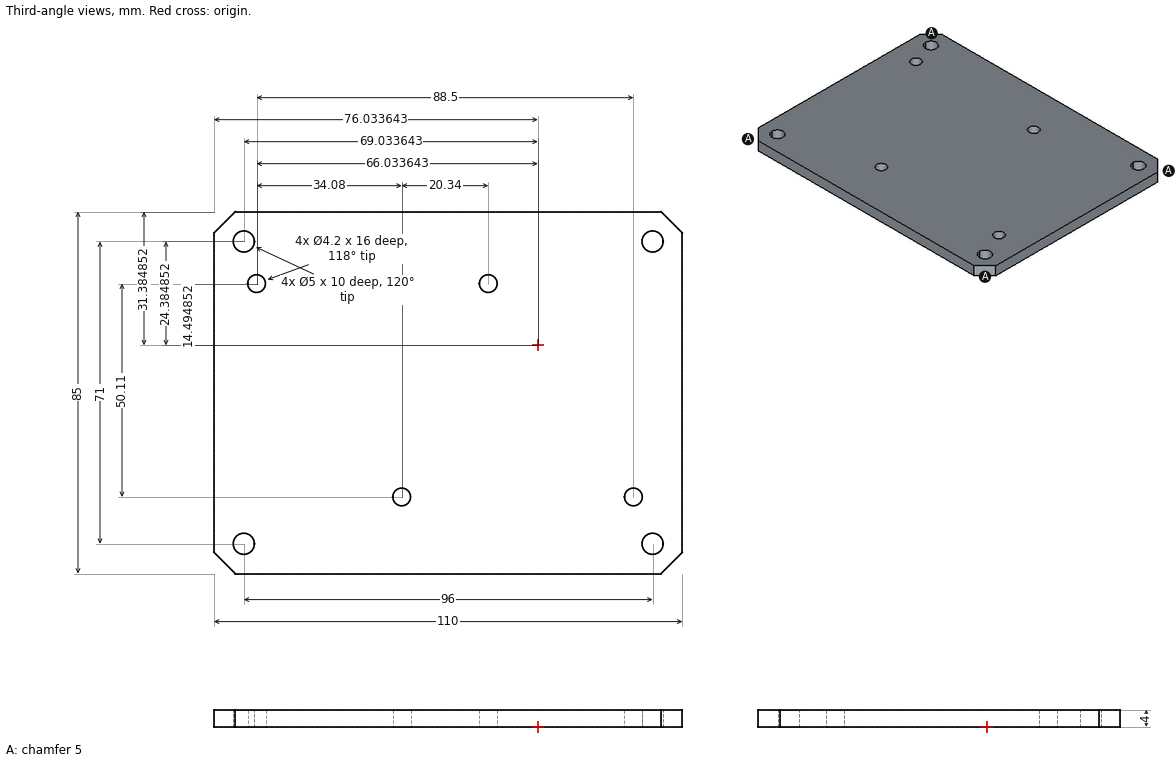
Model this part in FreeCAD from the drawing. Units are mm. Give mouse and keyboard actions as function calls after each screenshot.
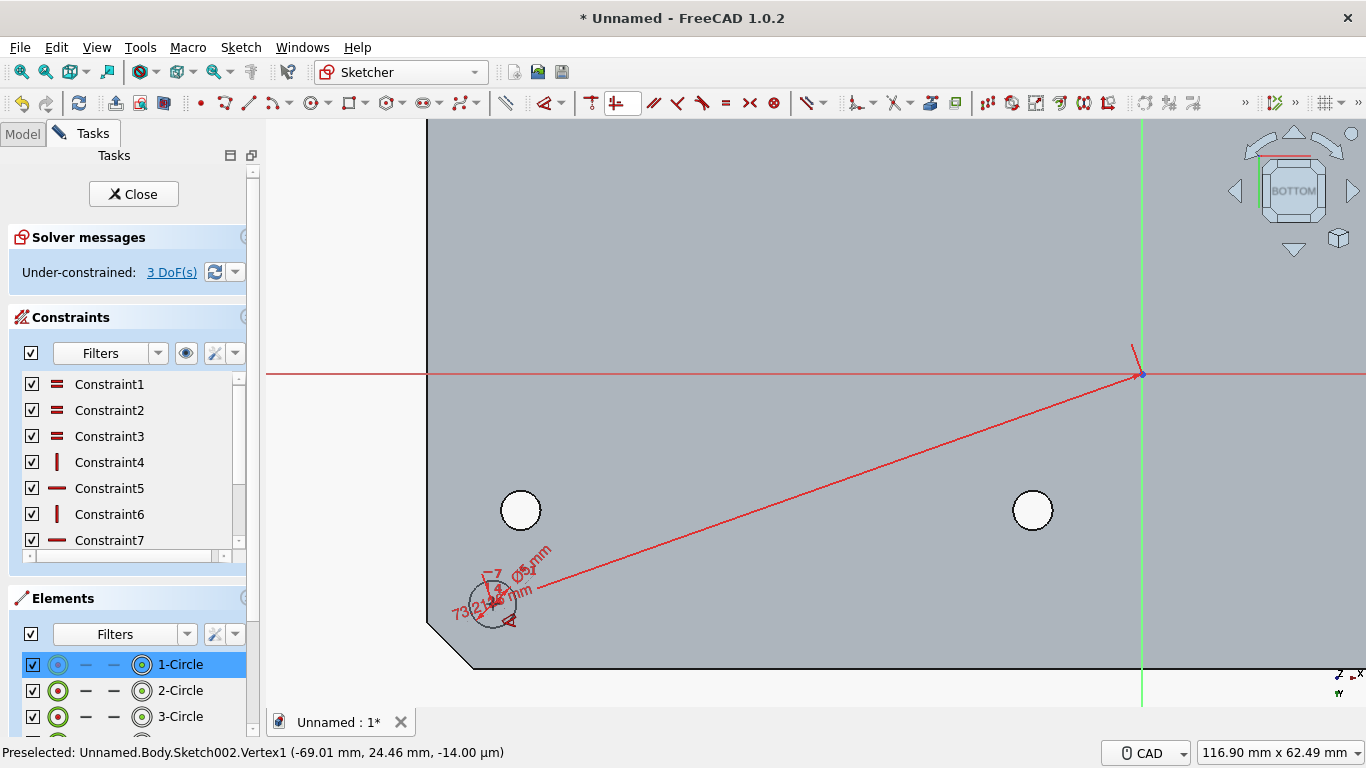
scroll(508, 588, down, 3)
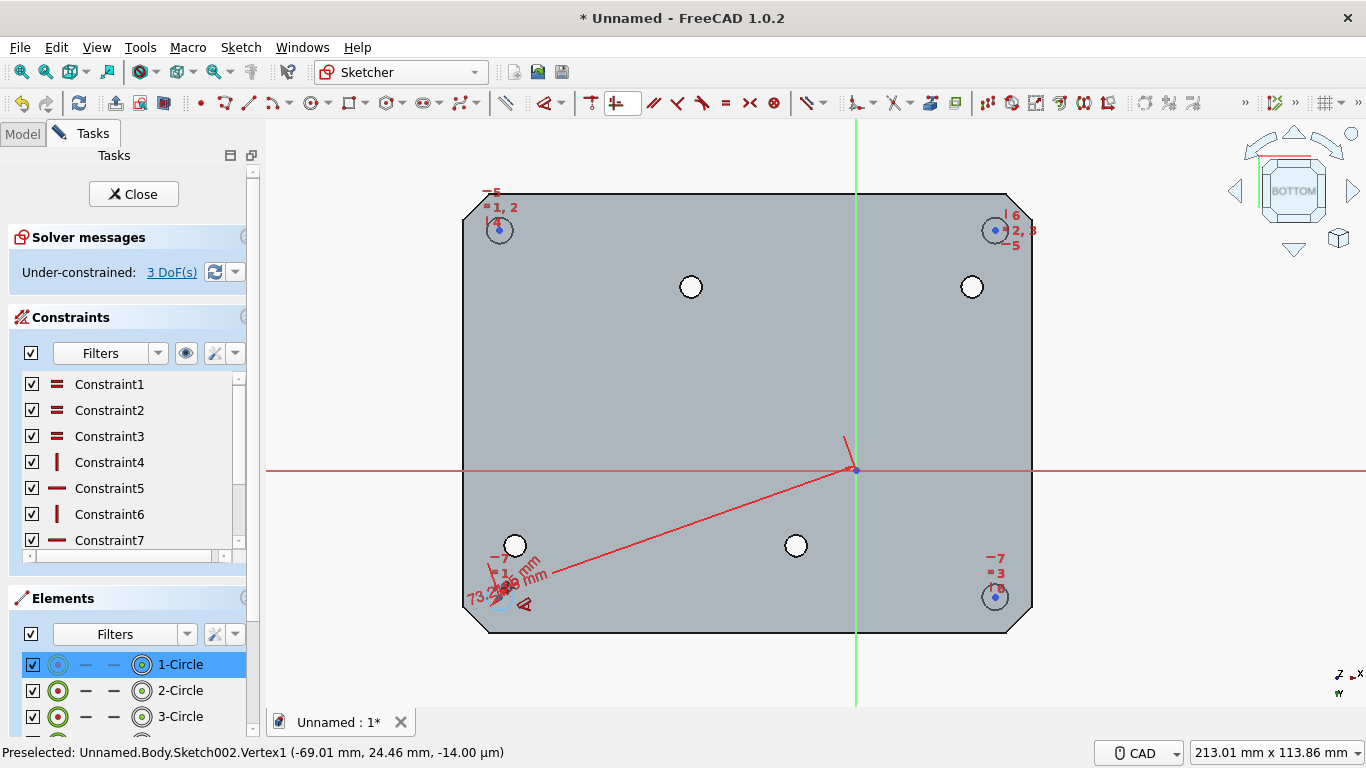
click(500, 231)
click(466, 414)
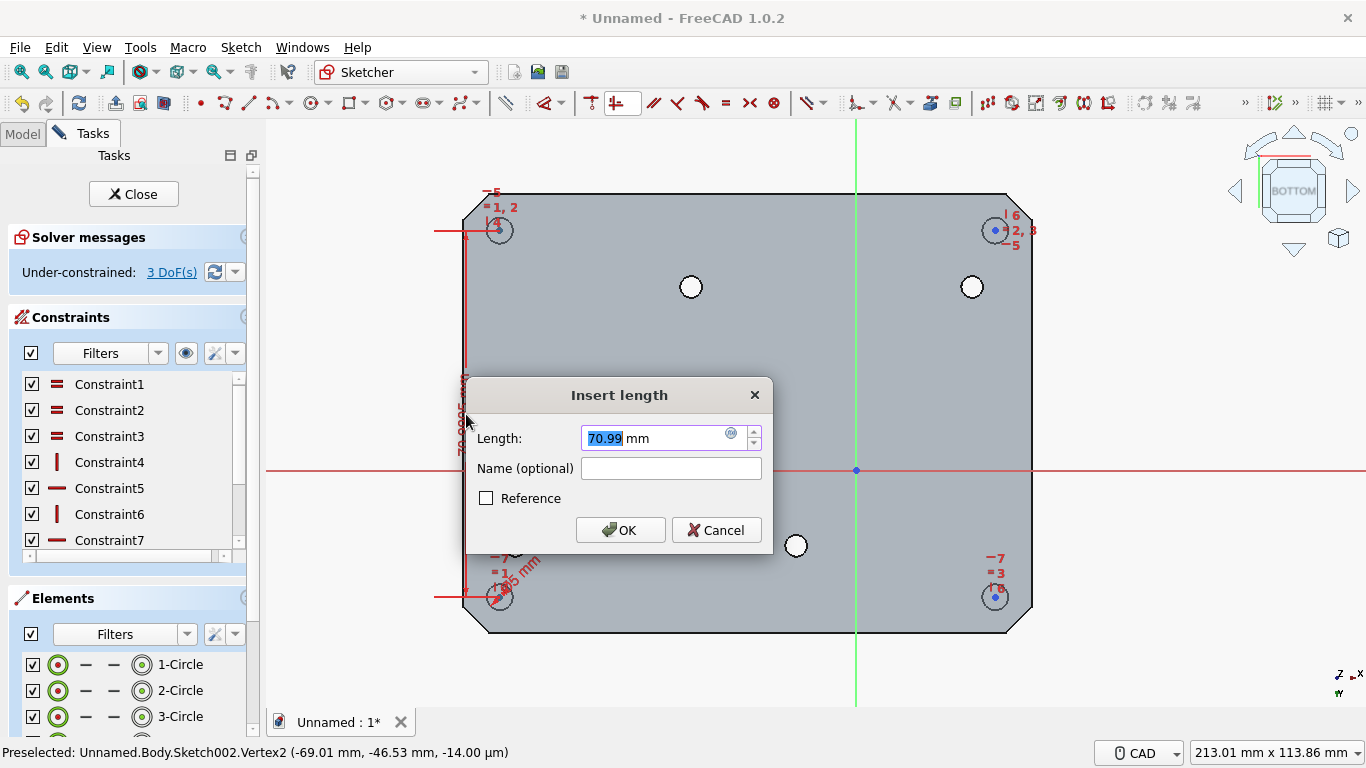
text(71)
key(Return)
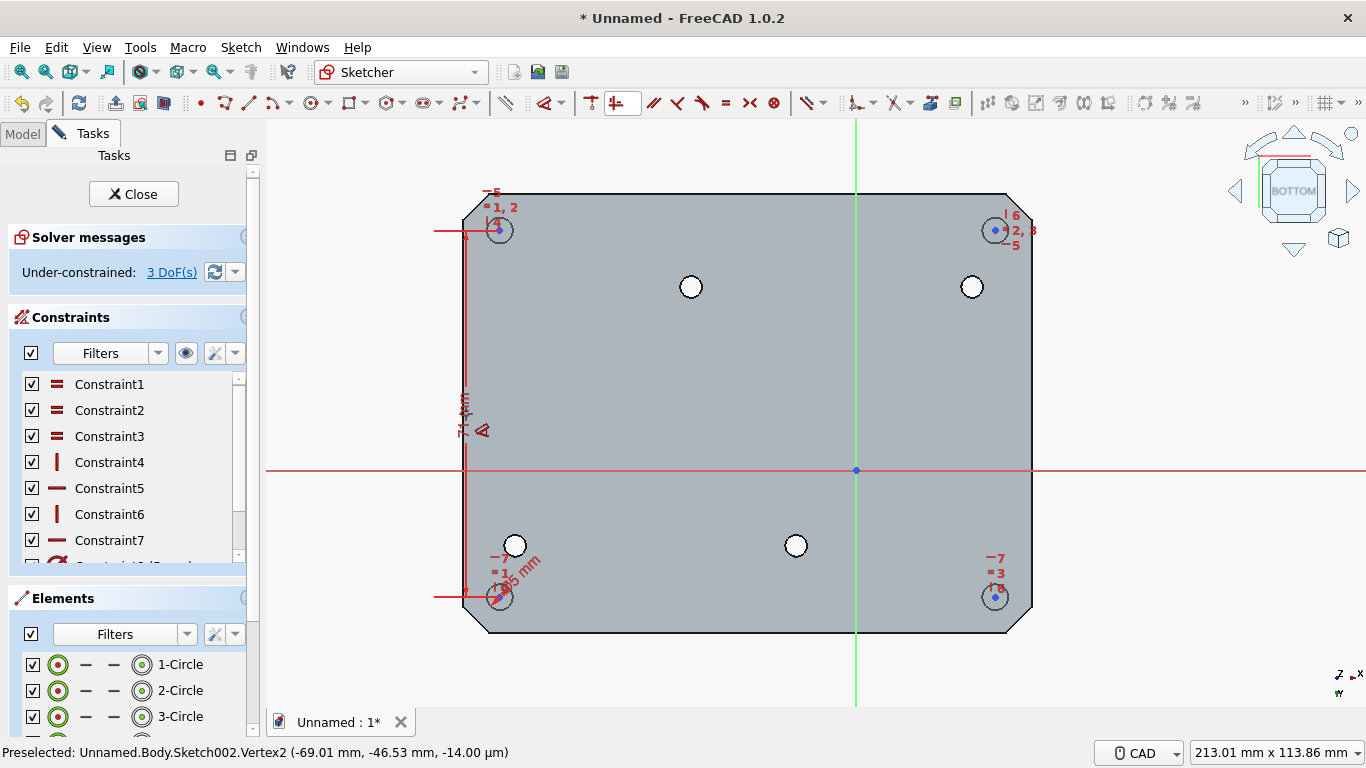
click(500, 231)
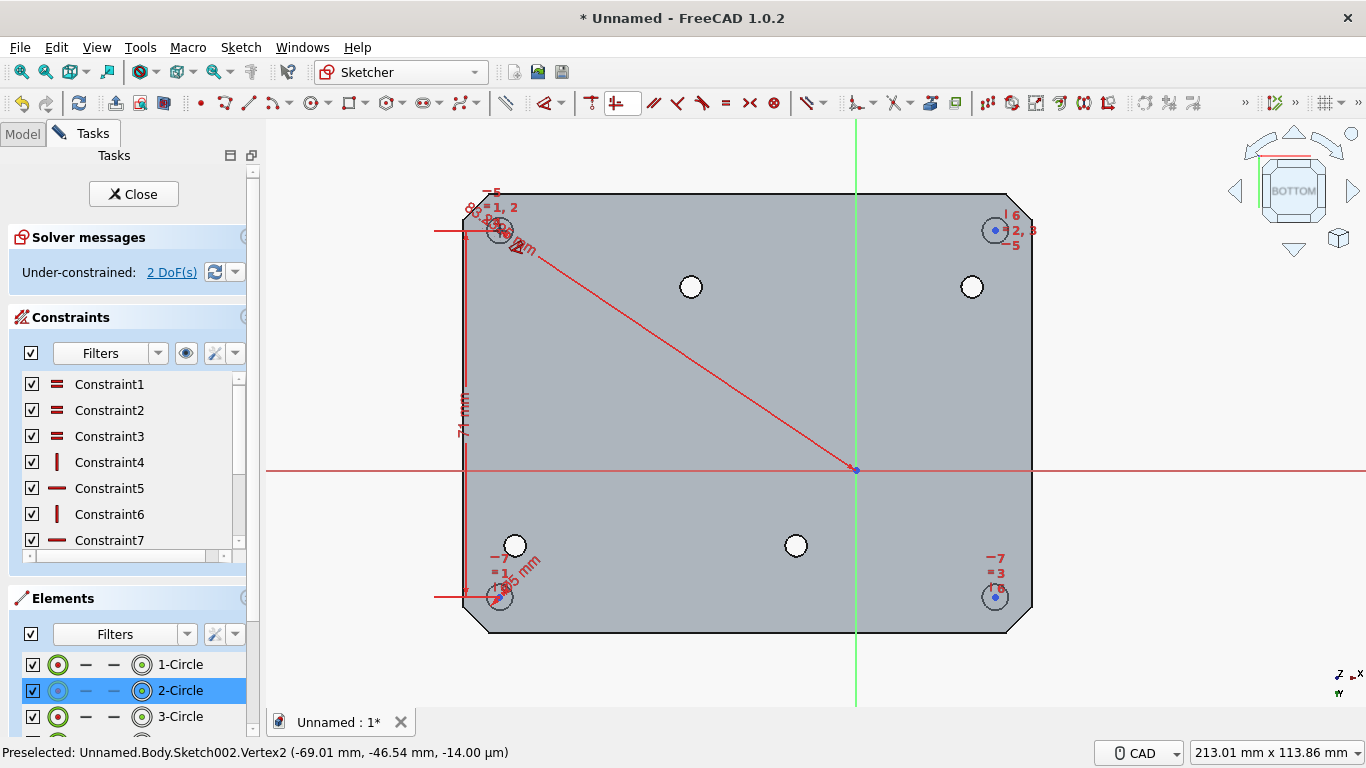
click(995, 231)
click(748, 197)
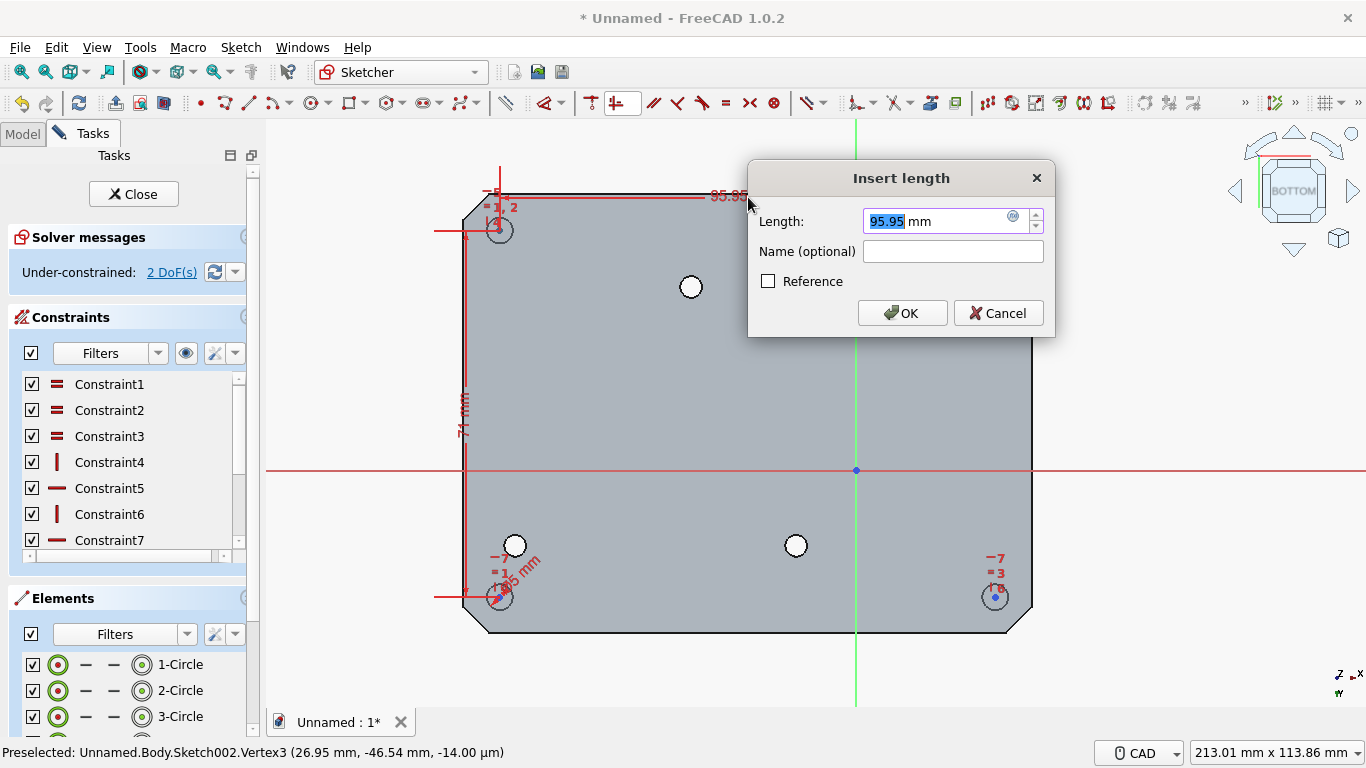
text(96)
key(Return)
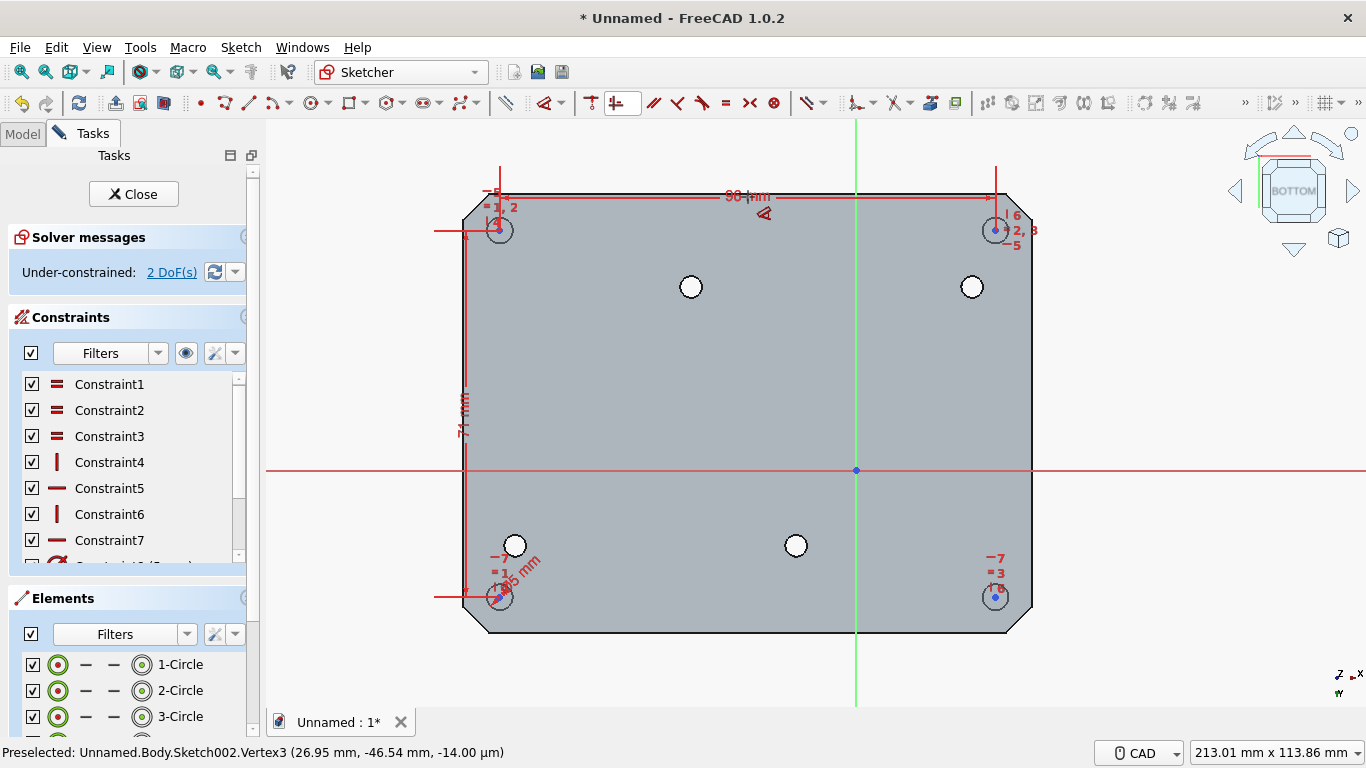
click(500, 597)
click(678, 631)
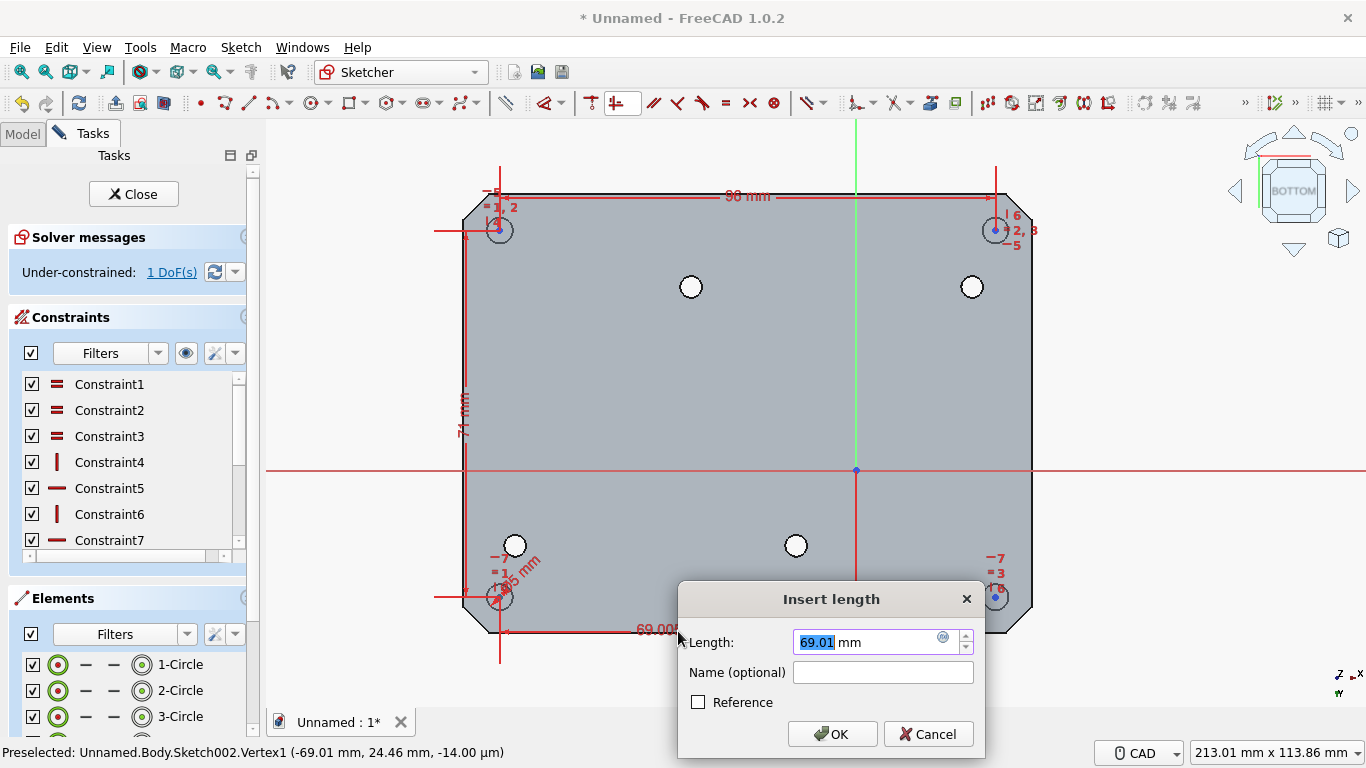
text(69.033643)
key(Return)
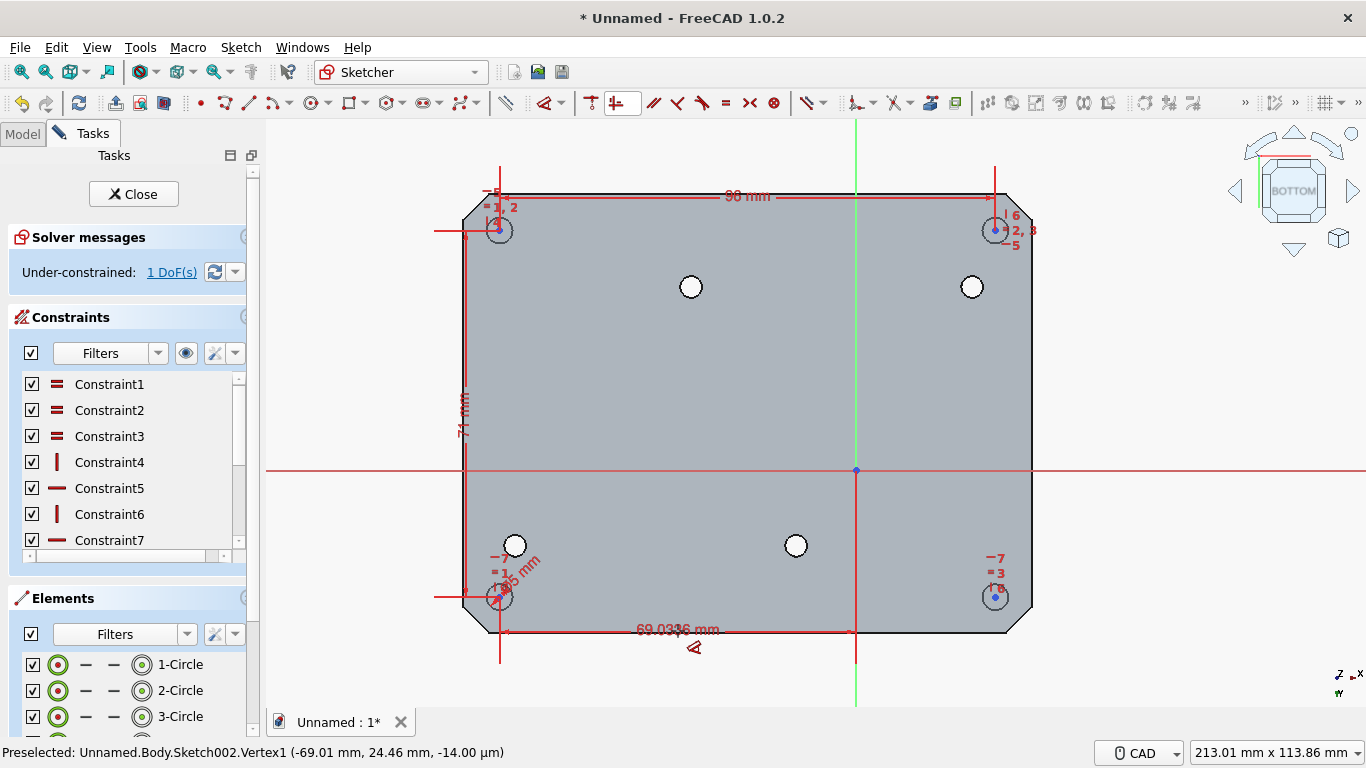
click(500, 597)
click(466, 534)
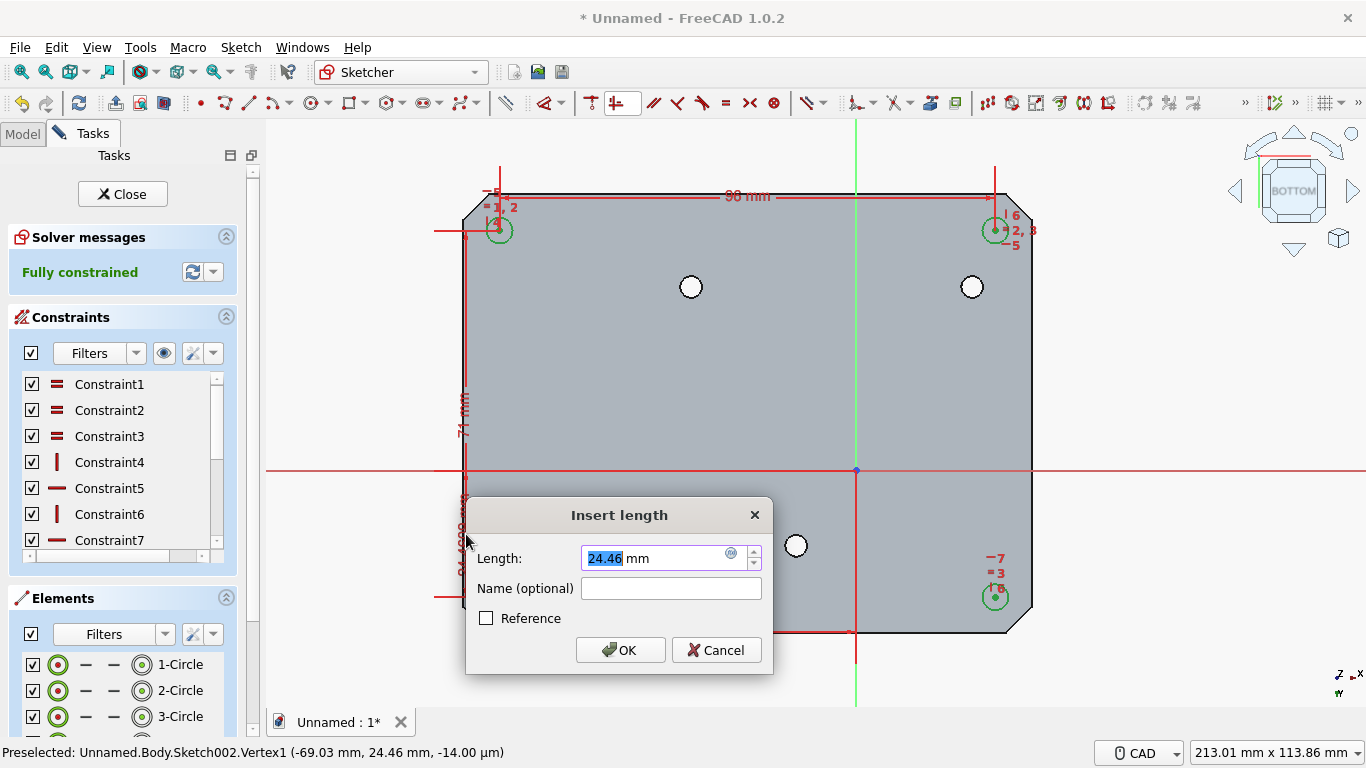
text(24.384852)
key(Return)
key(Escape)